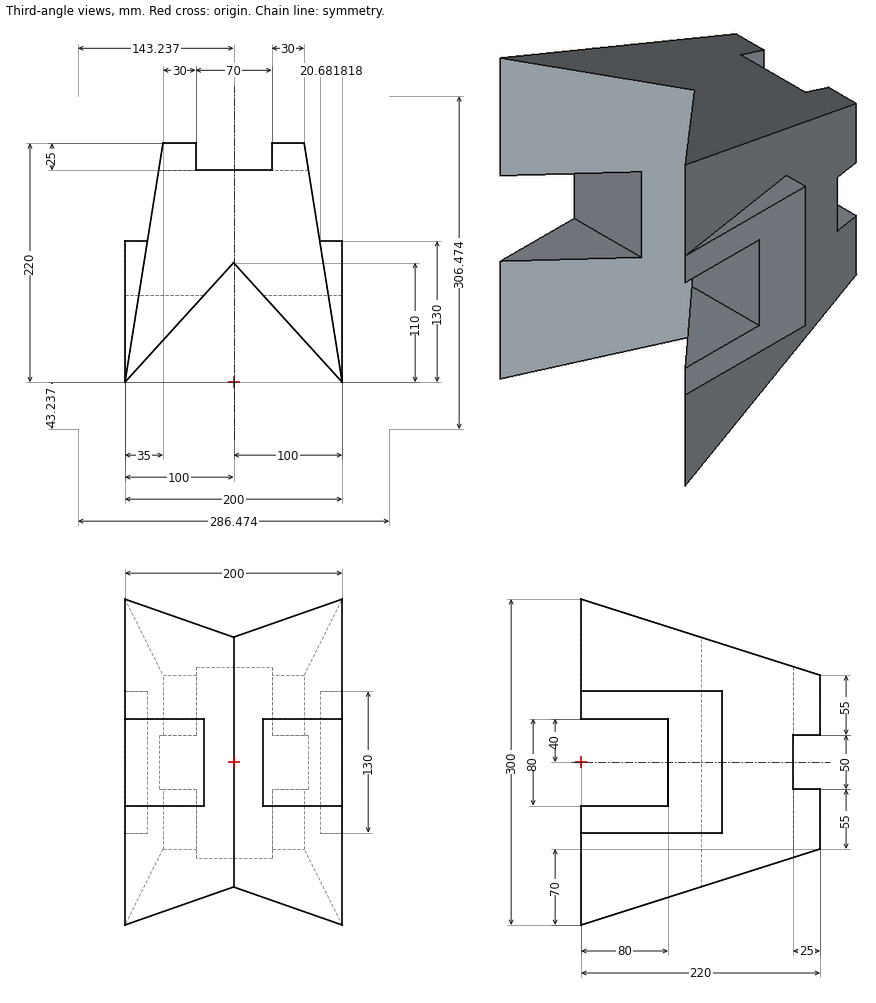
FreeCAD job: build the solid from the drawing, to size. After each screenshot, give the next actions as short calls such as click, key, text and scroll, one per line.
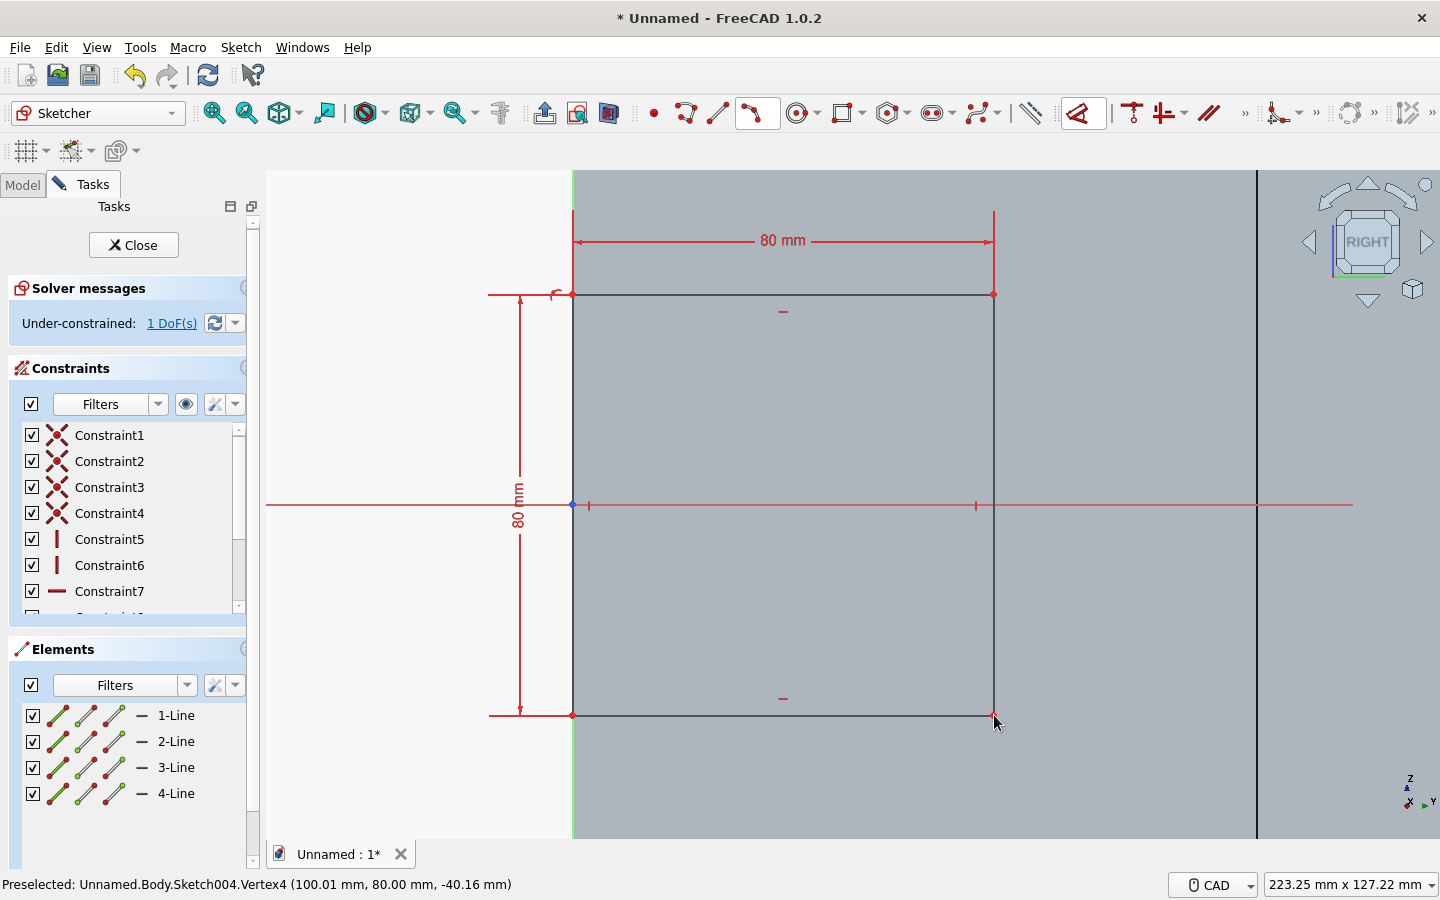
click(573, 295)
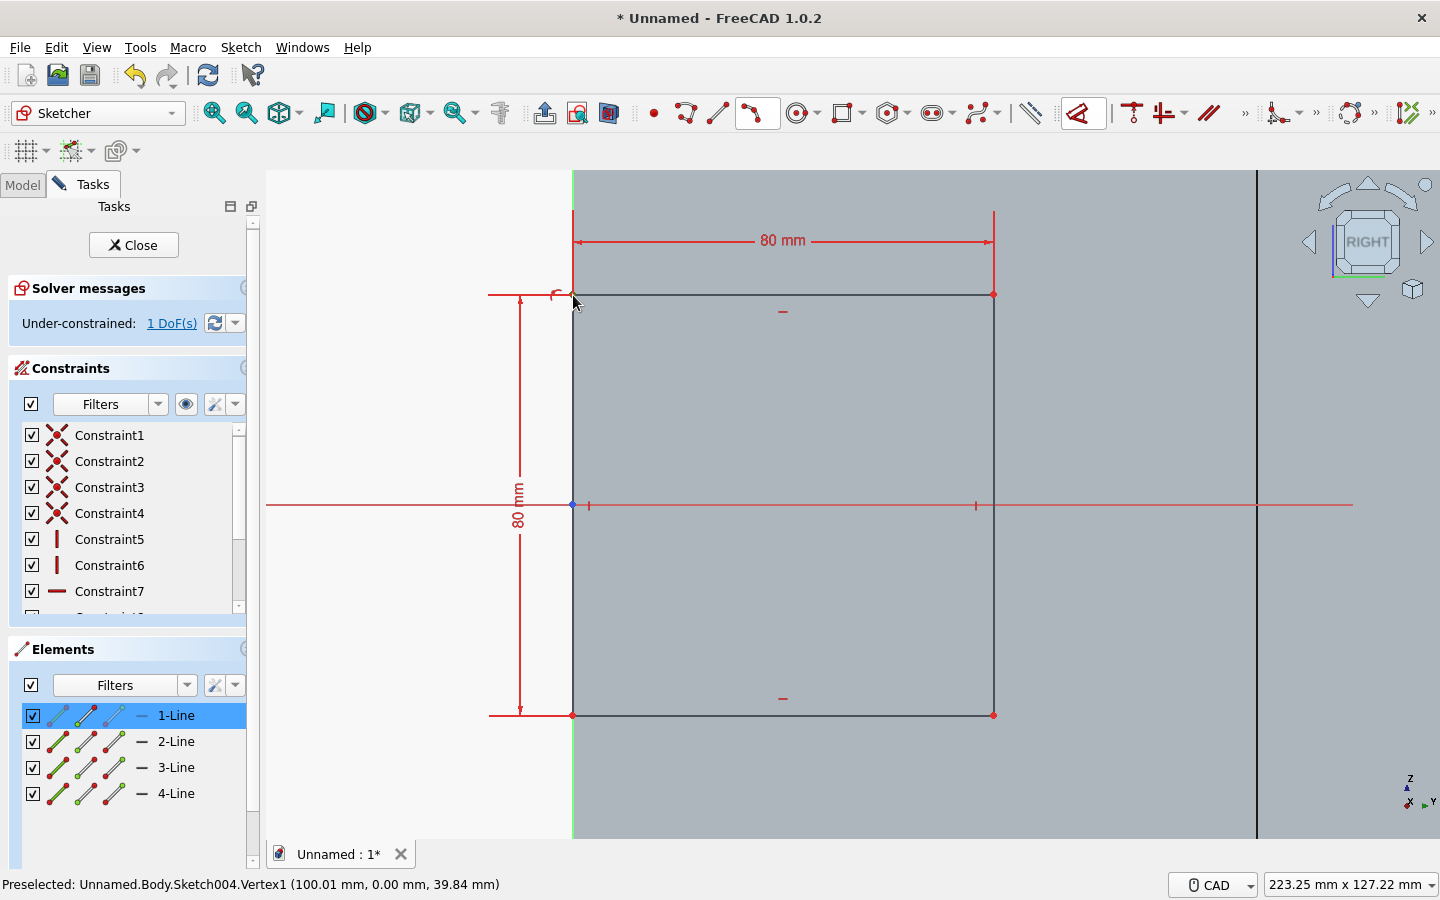
key(i)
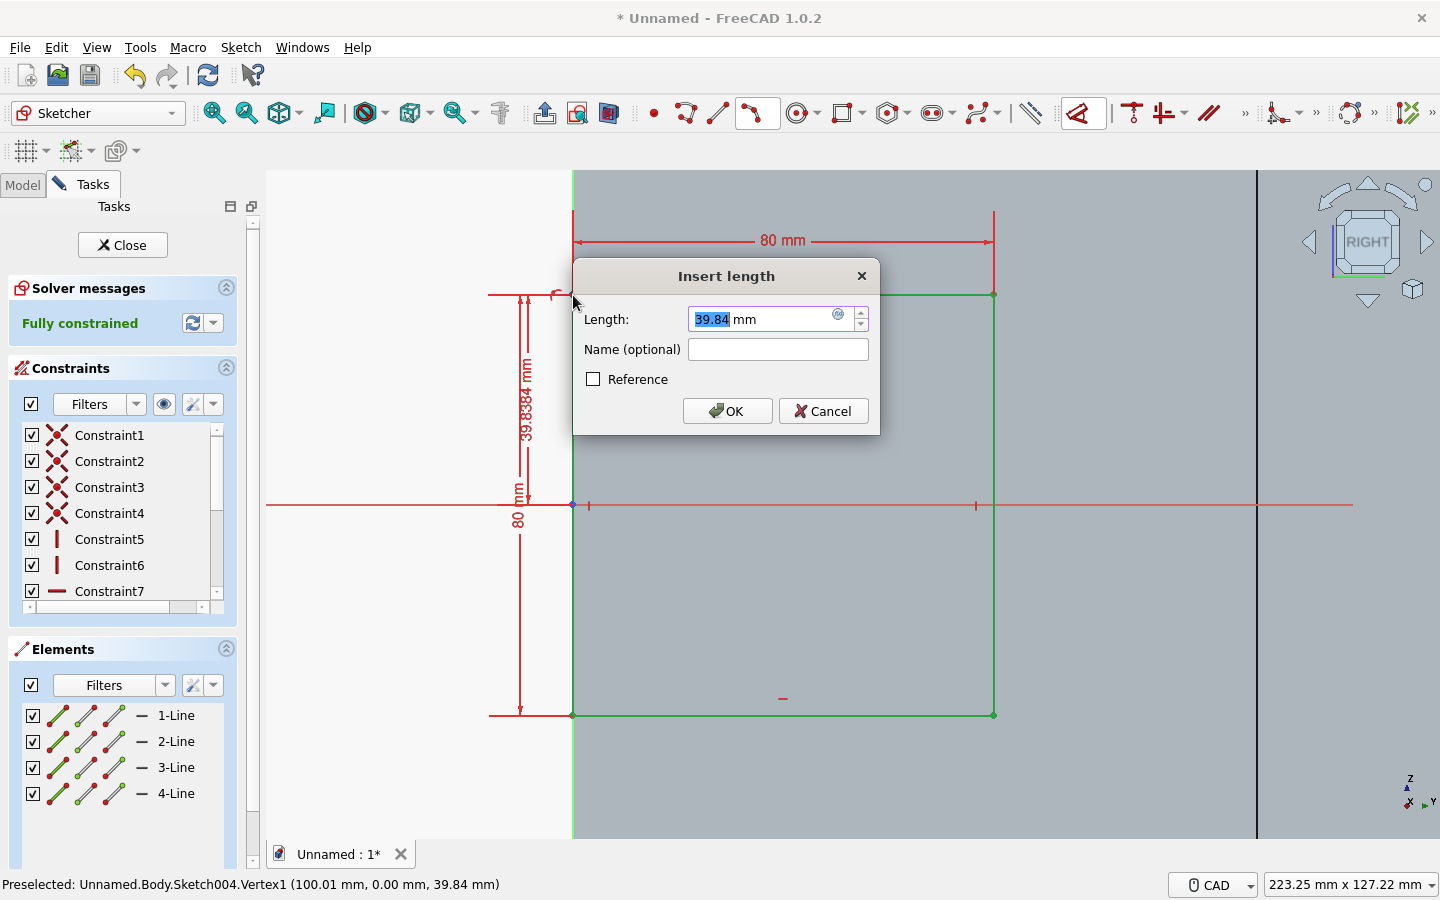
text(40)
key(Return)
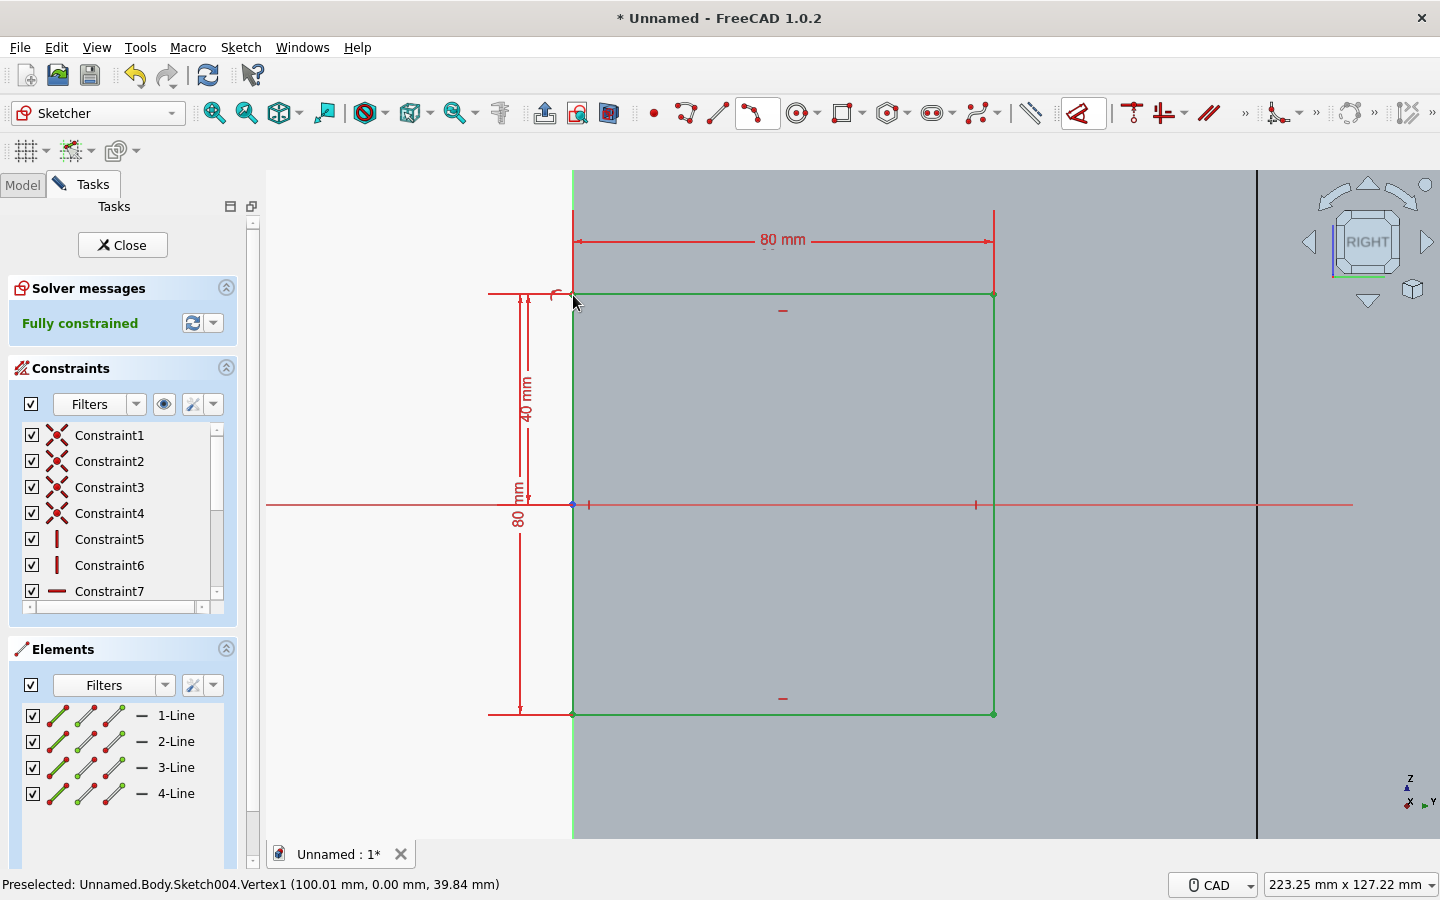
click(123, 245)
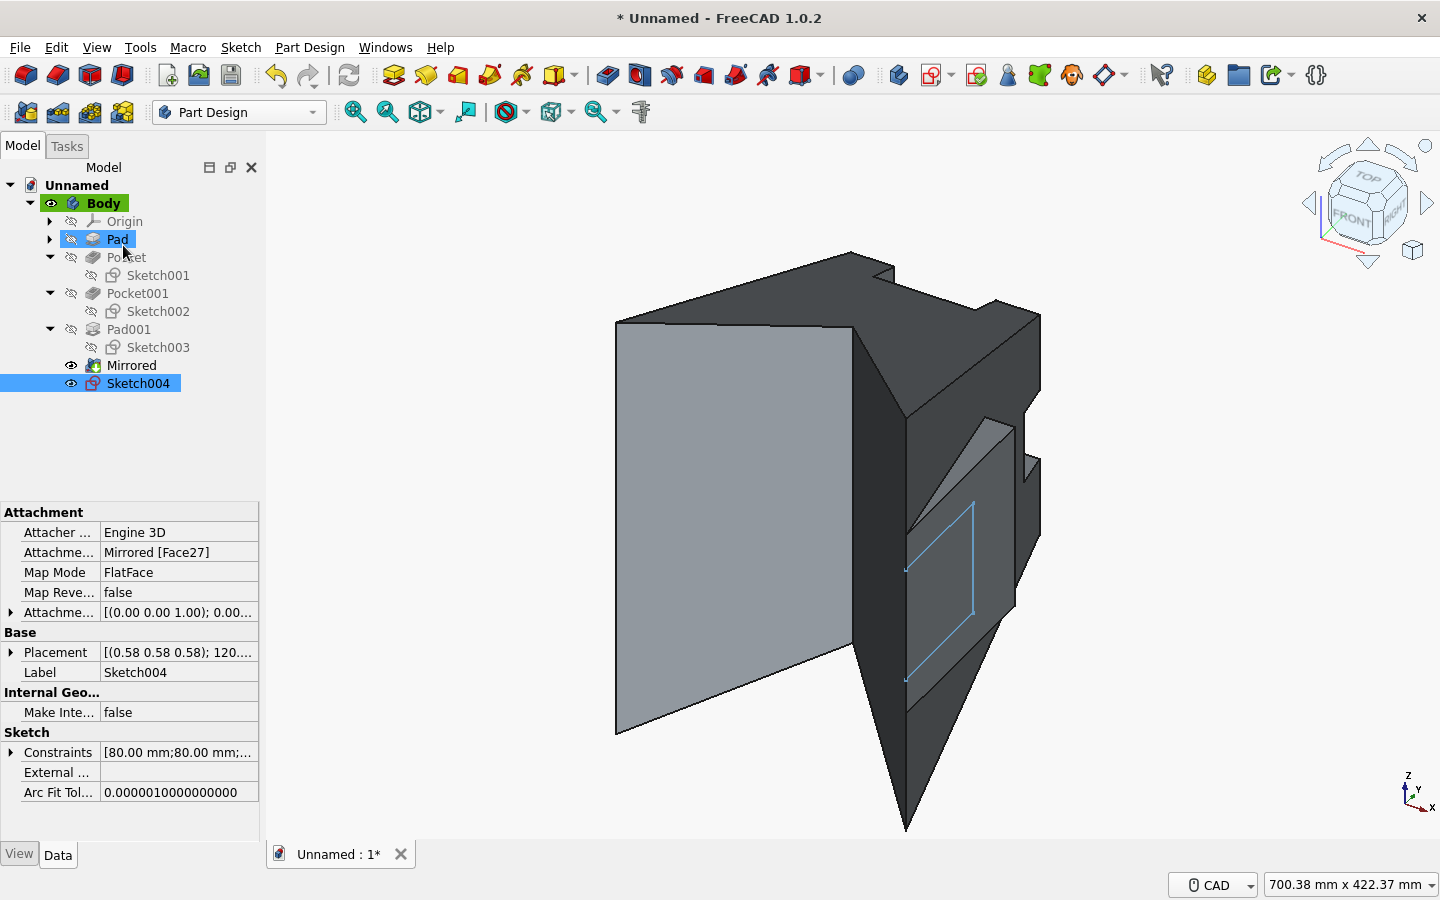
click(608, 76)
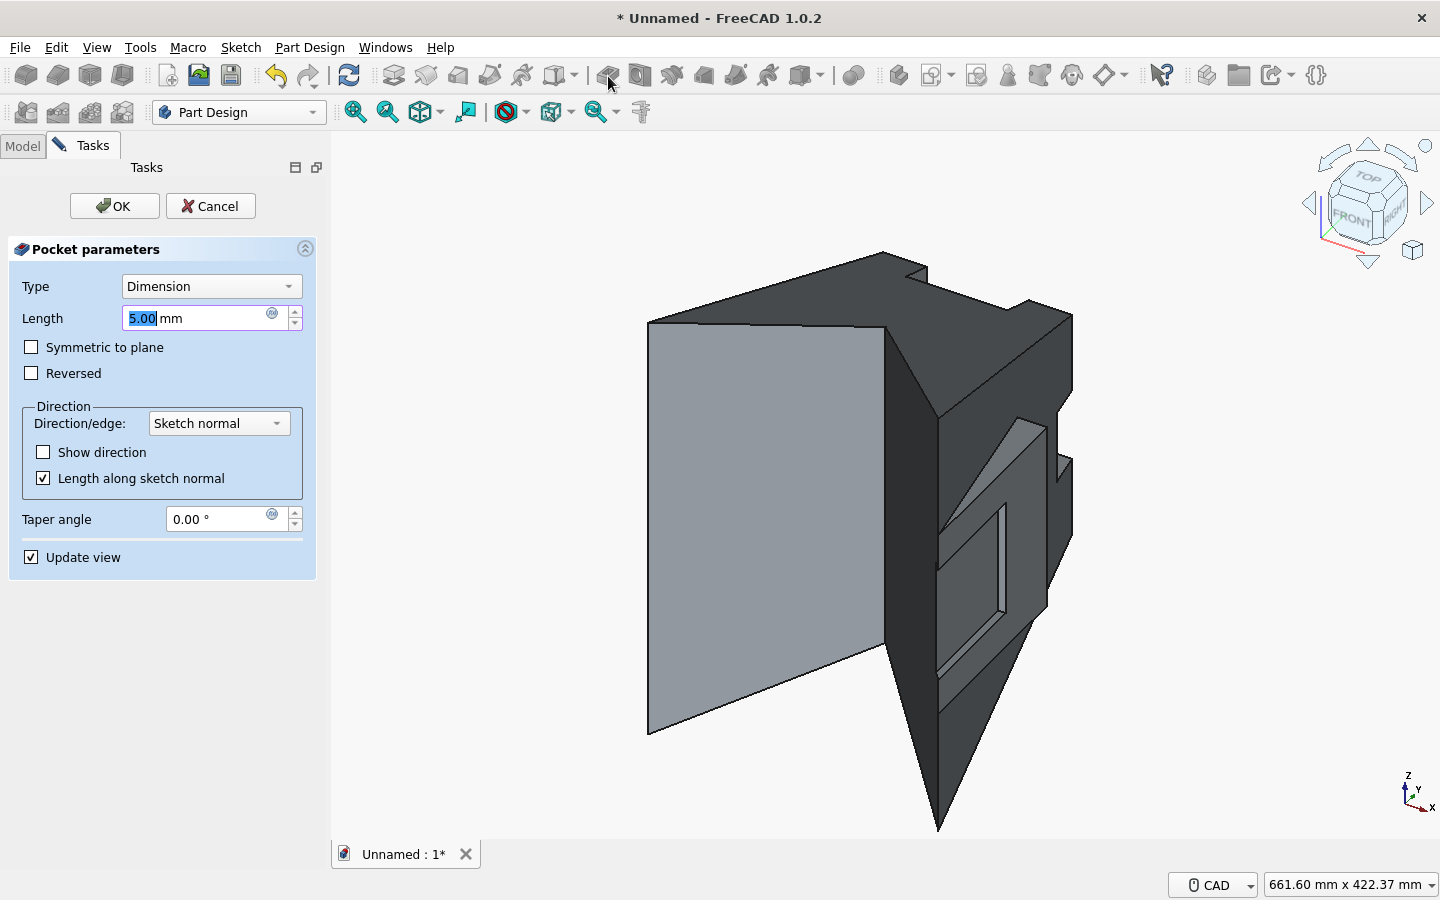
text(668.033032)
key(Tab)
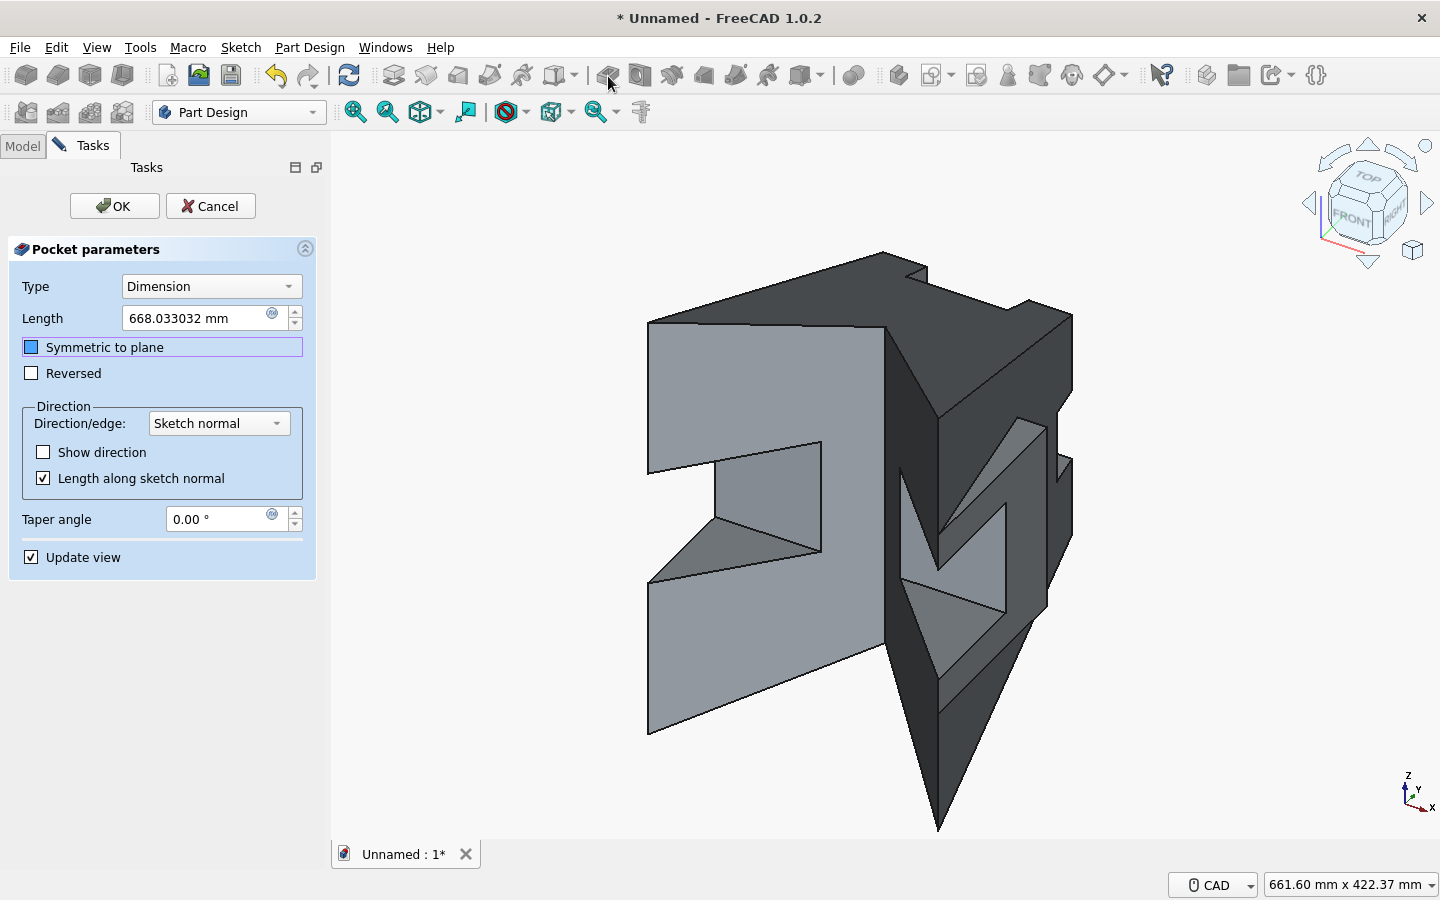
click(30, 347)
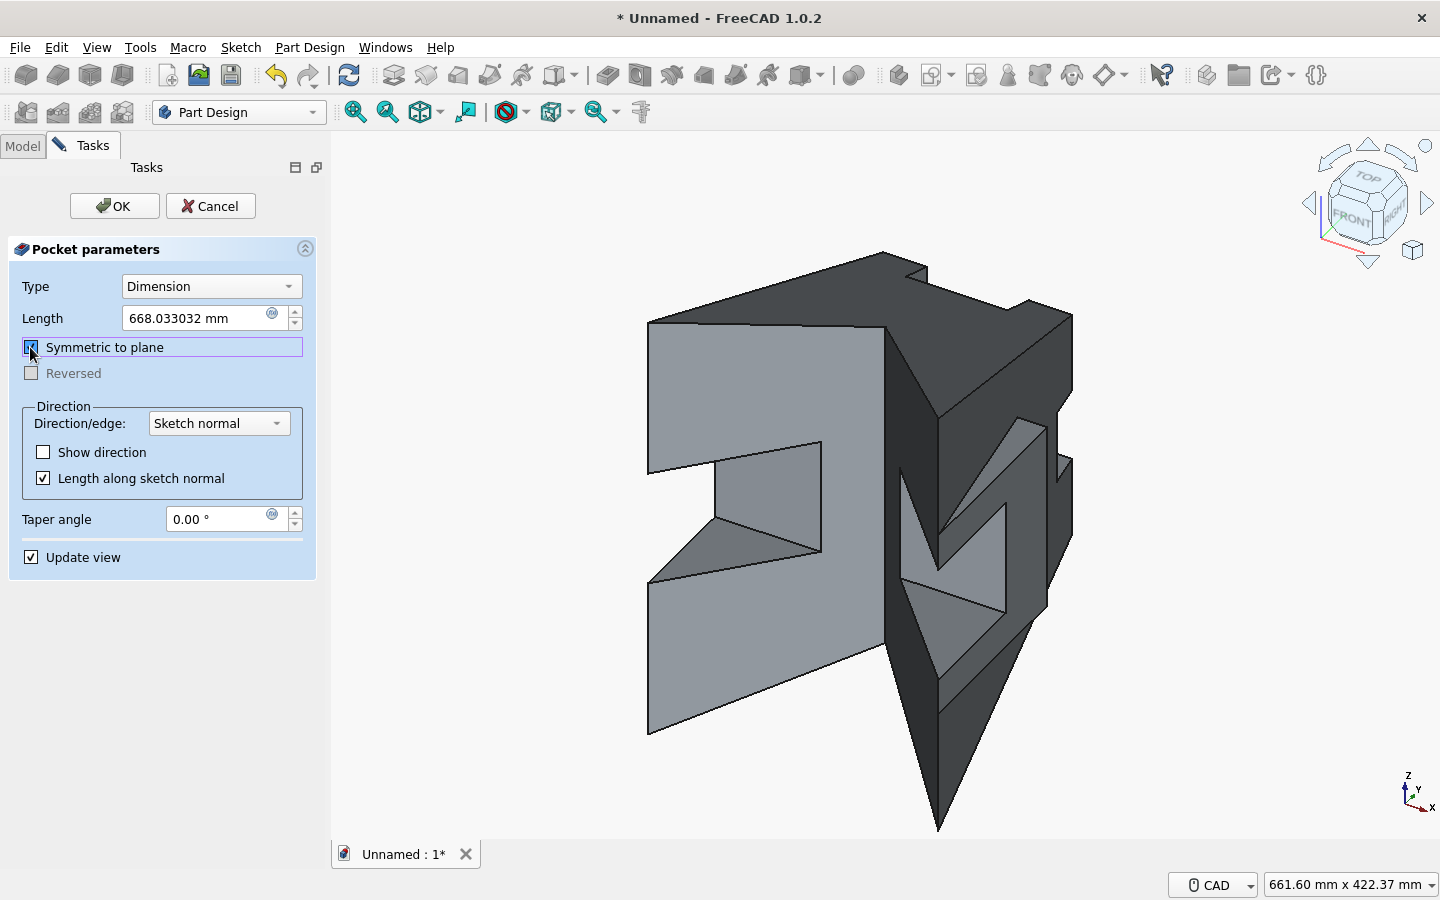
click(115, 206)